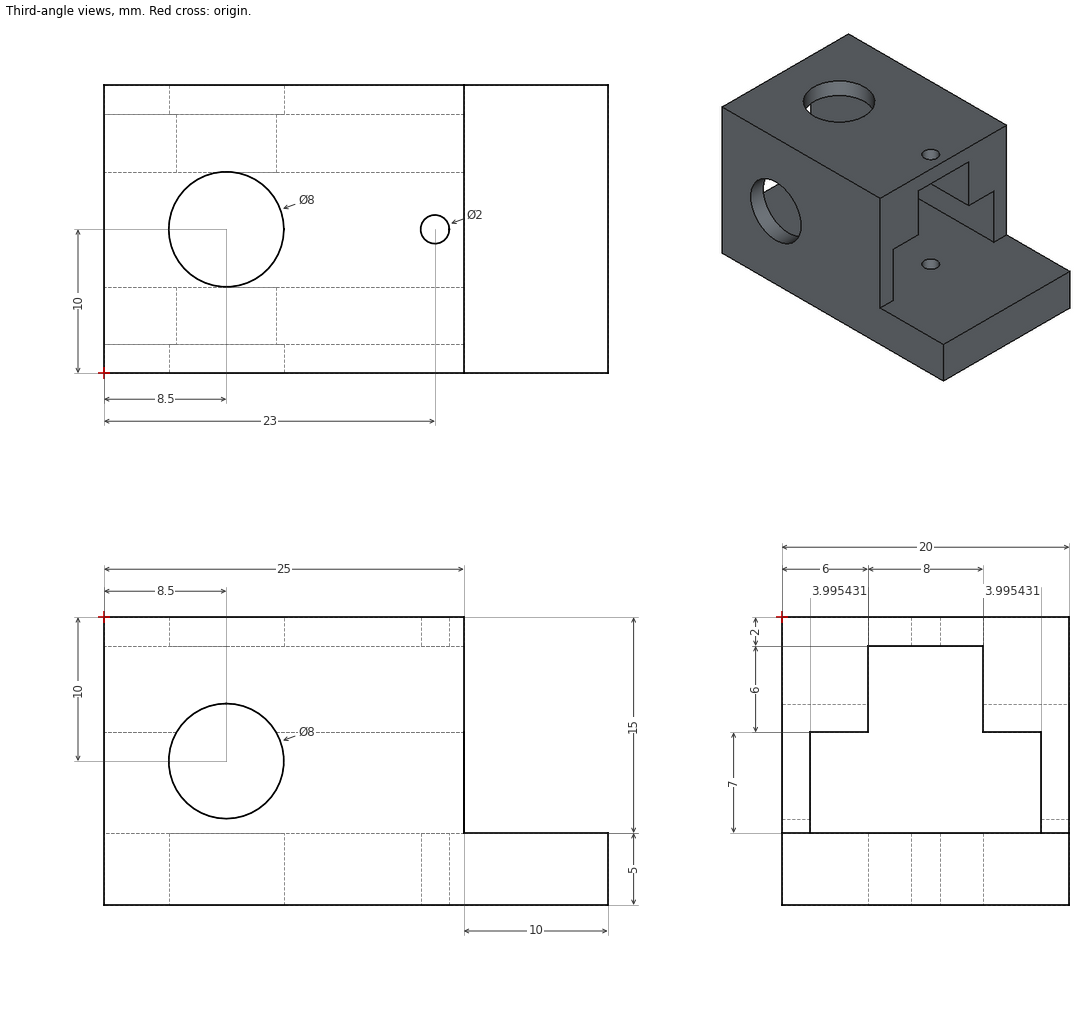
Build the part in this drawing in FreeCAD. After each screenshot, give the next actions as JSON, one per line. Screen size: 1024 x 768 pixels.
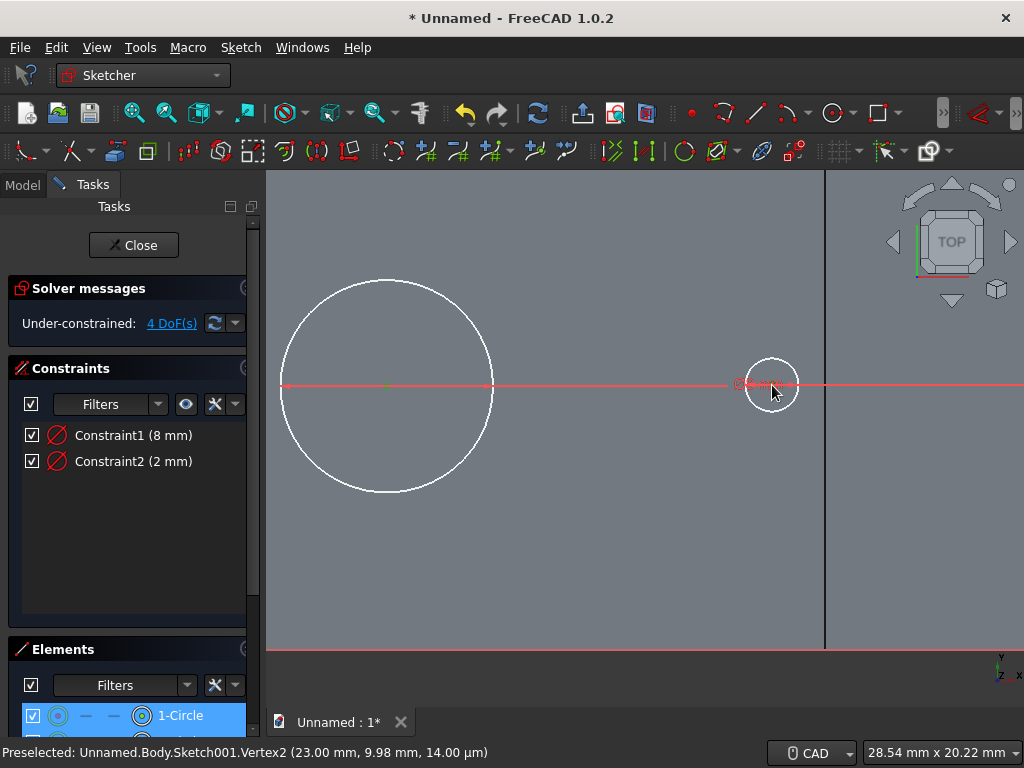
{"action": "key", "text": "h"}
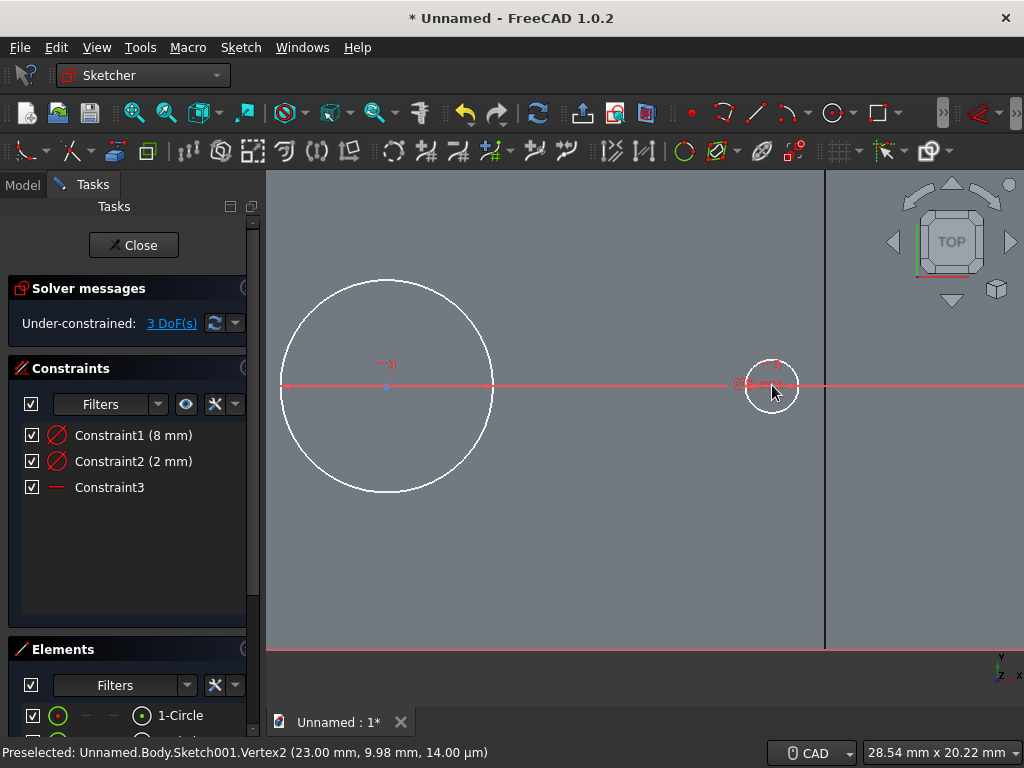
{"action": "left_click", "coordinate": [978, 114]}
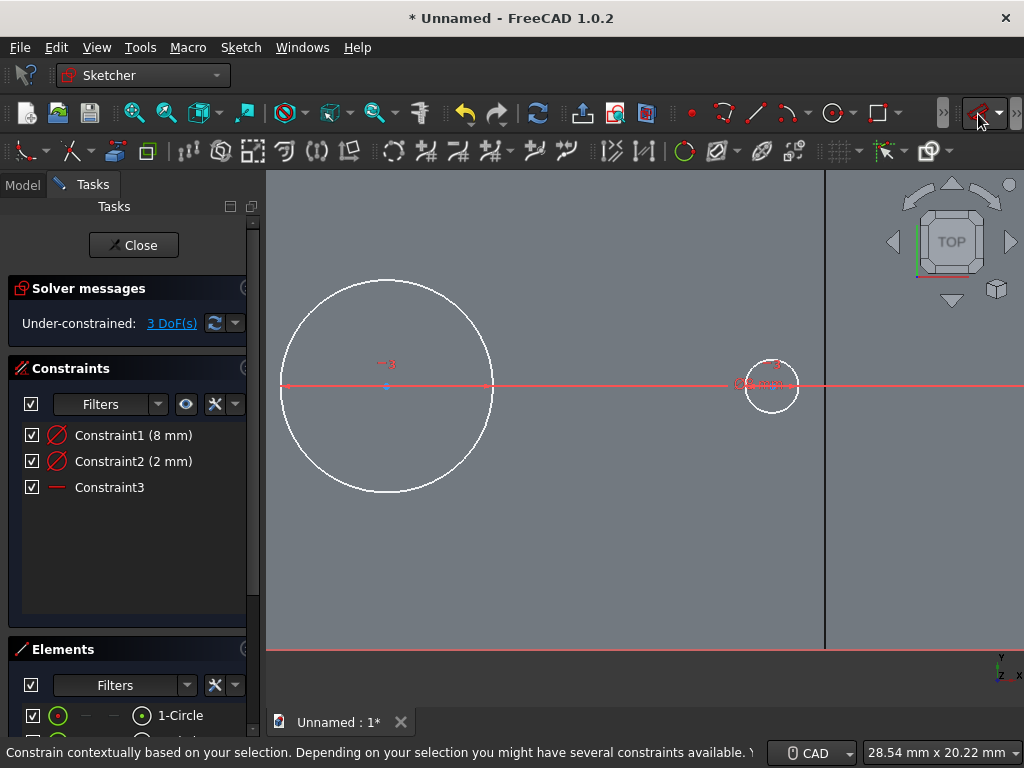
{"action": "left_click", "coordinate": [387, 386]}
{"action": "left_click", "coordinate": [421, 518]}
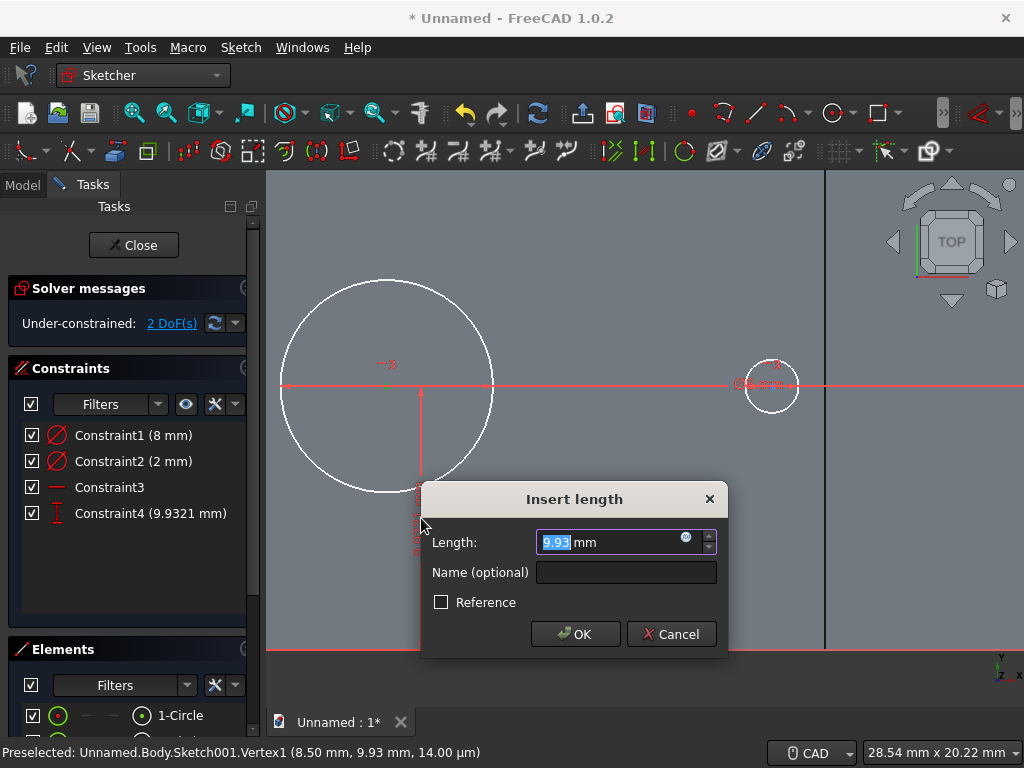
{"action": "type", "text": "10"}
{"action": "key", "text": "Return"}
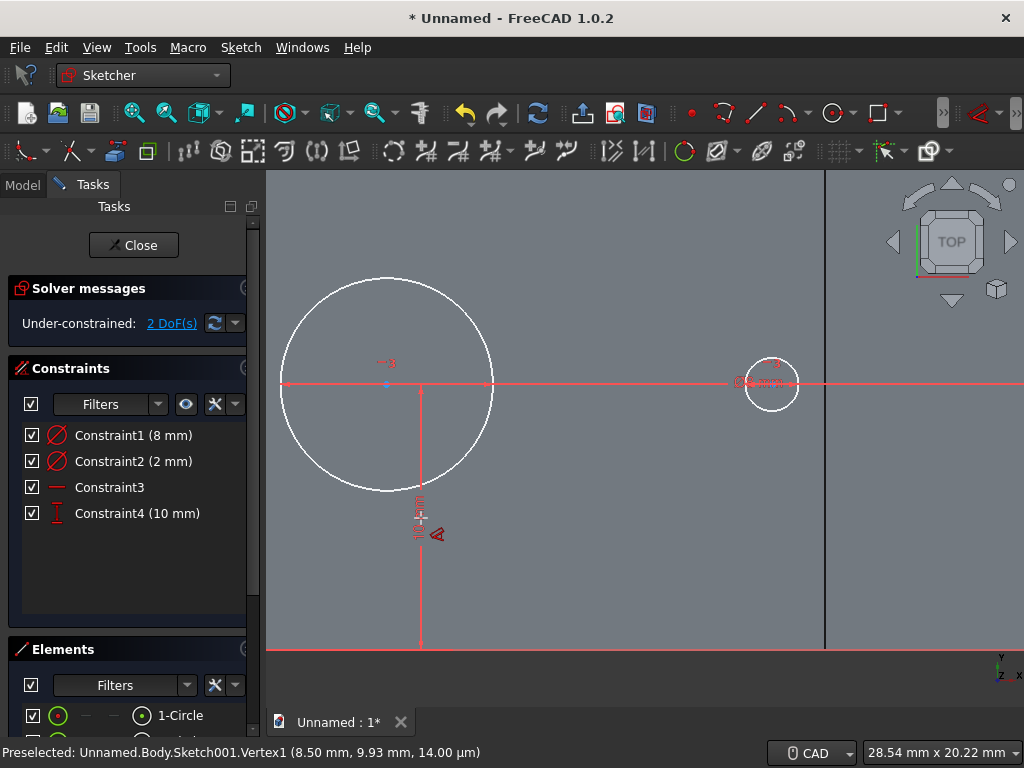
{"action": "left_click", "coordinate": [772, 384]}
{"action": "left_click", "coordinate": [533, 350]}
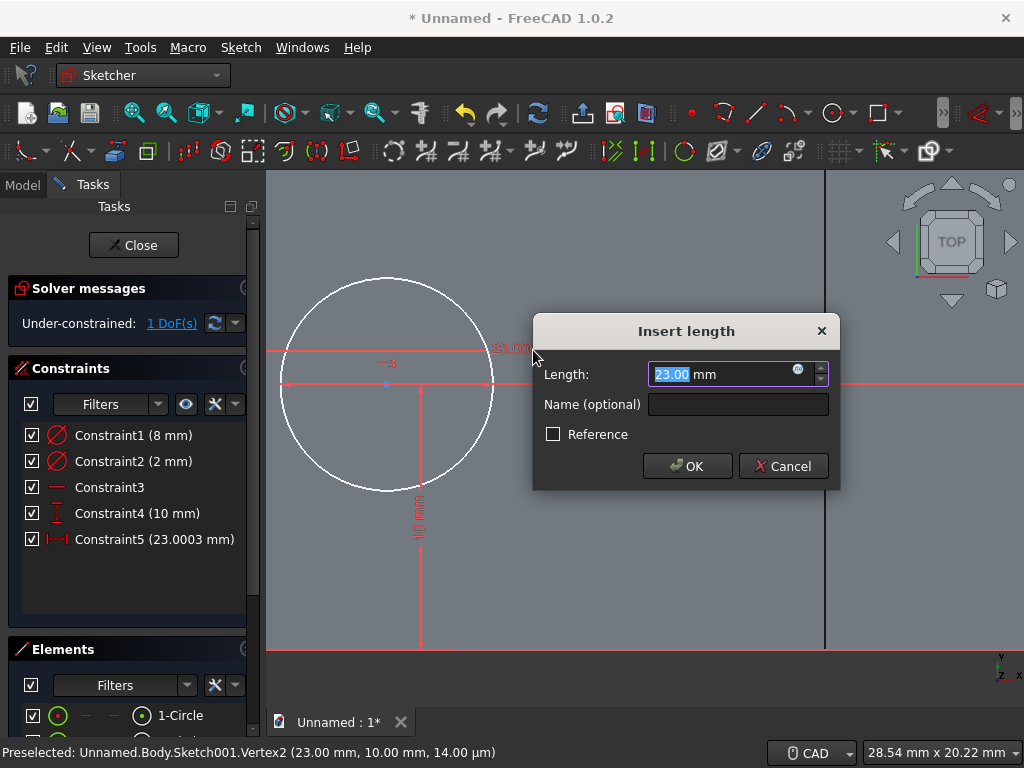
{"action": "type", "text": "23"}
{"action": "key", "text": "Return"}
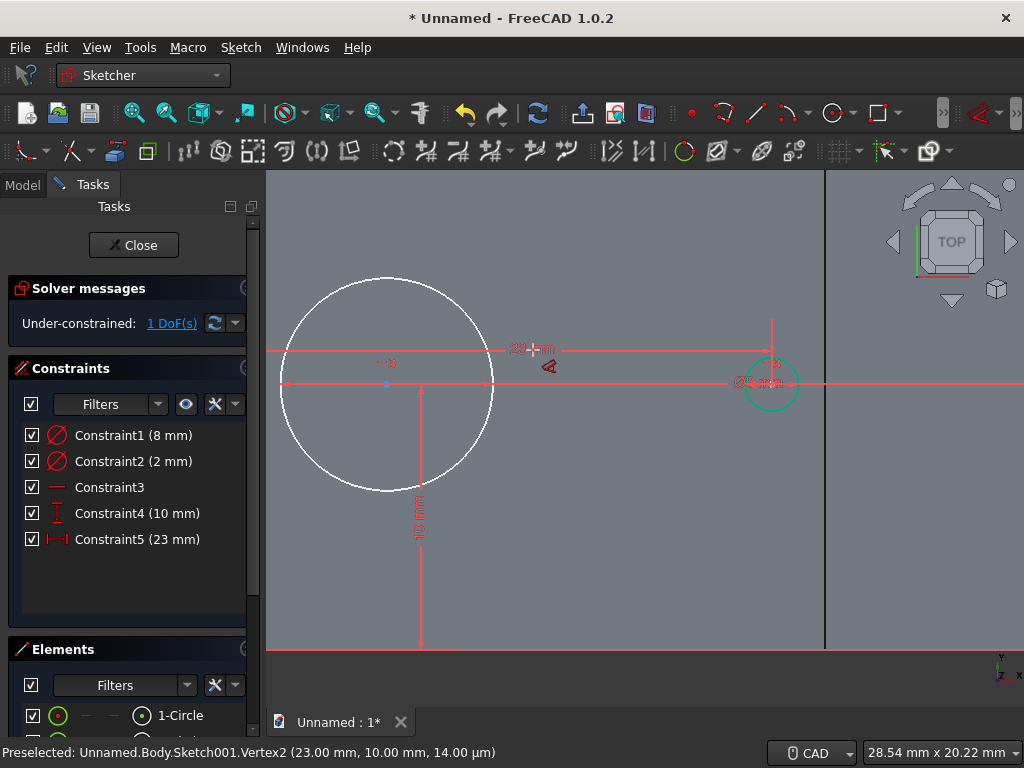
{"action": "left_click", "coordinate": [387, 384]}
{"action": "left_click", "coordinate": [340, 350]}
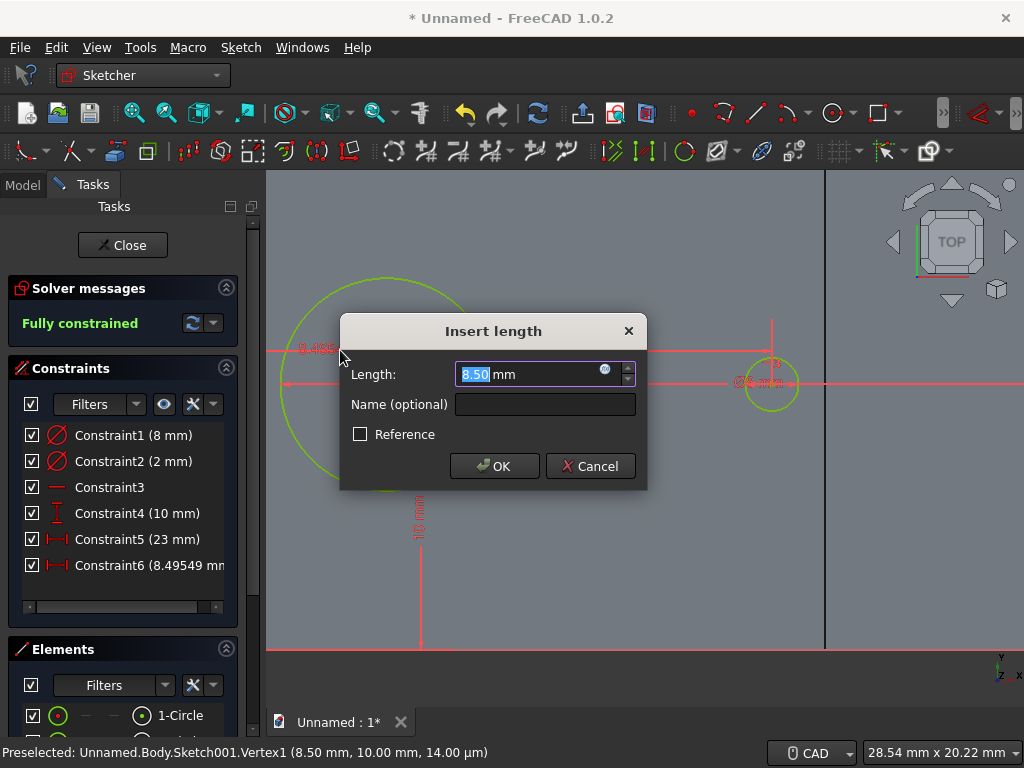
{"action": "type", "text": "8.5"}
{"action": "key", "text": "Return"}
{"action": "key", "text": "Escape"}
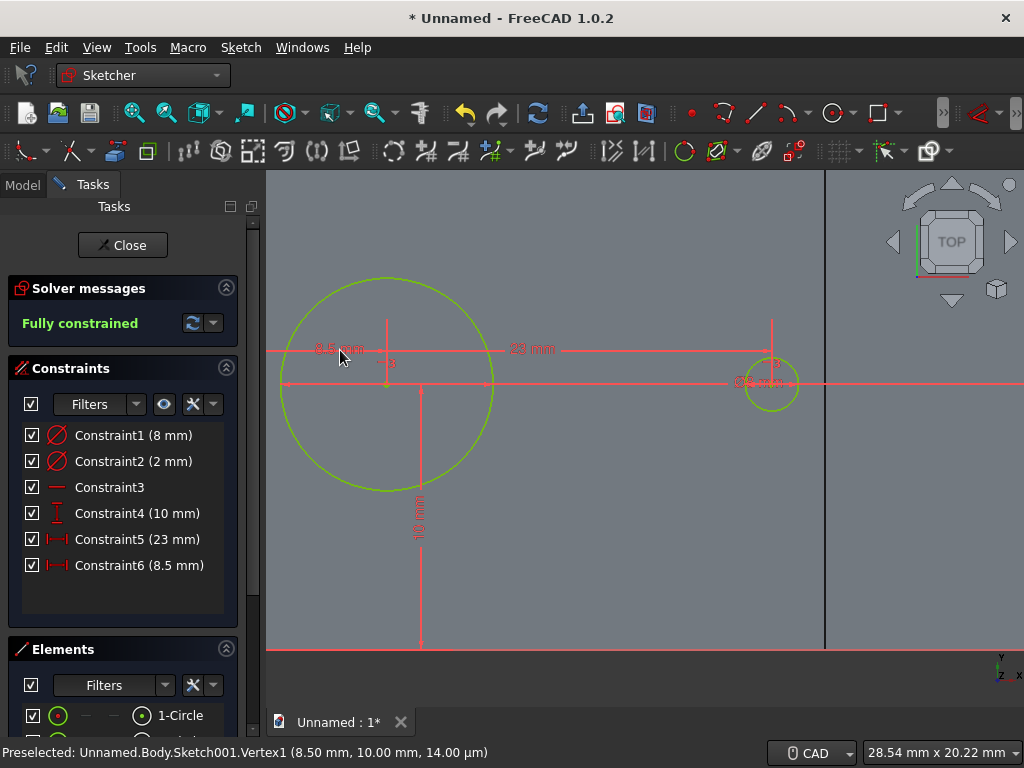
{"action": "left_click", "coordinate": [123, 245]}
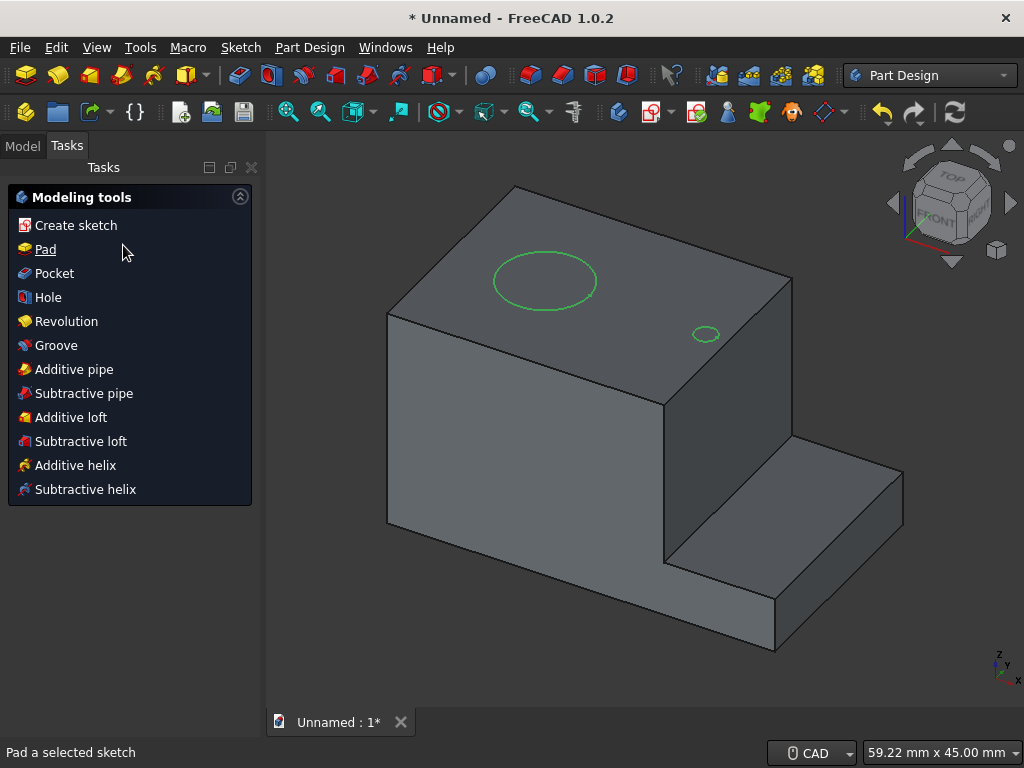
{"action": "left_click", "coordinate": [240, 76]}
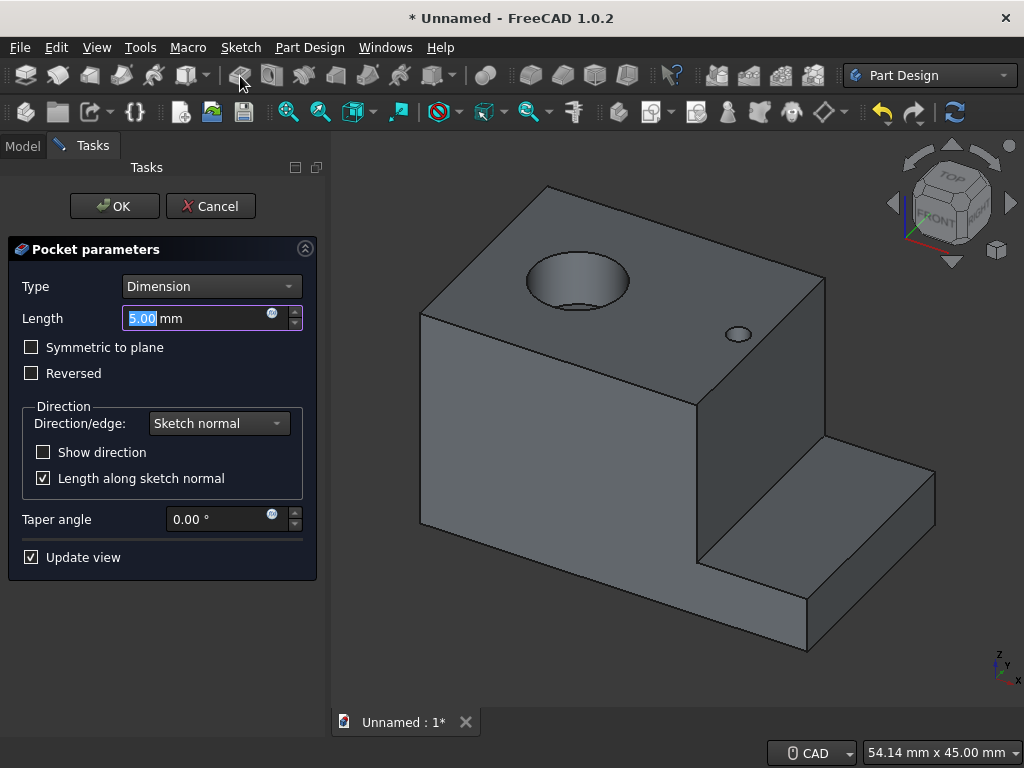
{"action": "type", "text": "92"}
{"action": "key", "text": "Tab"}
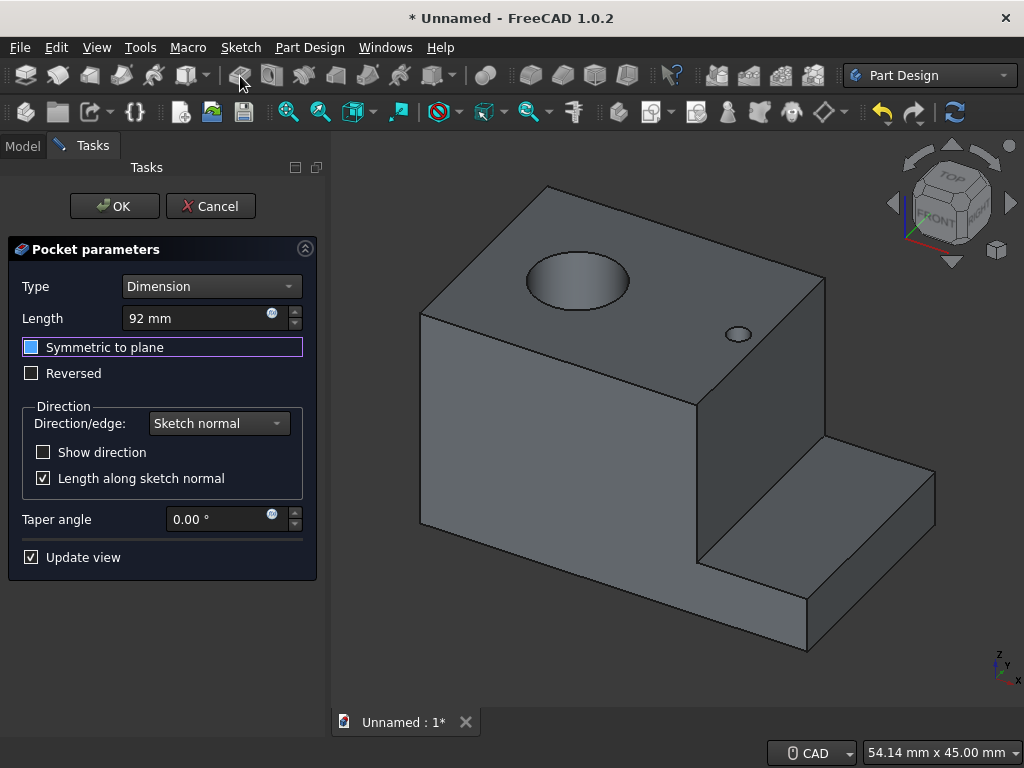
{"action": "left_click", "coordinate": [30, 347]}